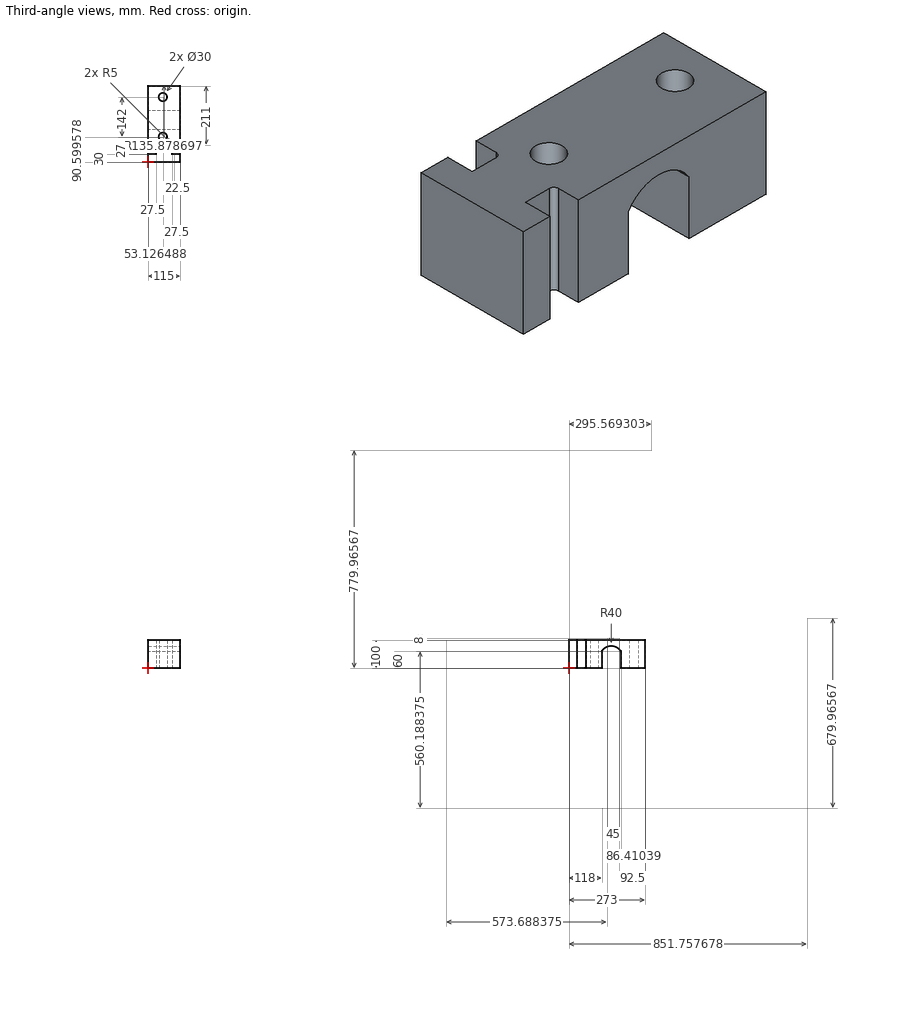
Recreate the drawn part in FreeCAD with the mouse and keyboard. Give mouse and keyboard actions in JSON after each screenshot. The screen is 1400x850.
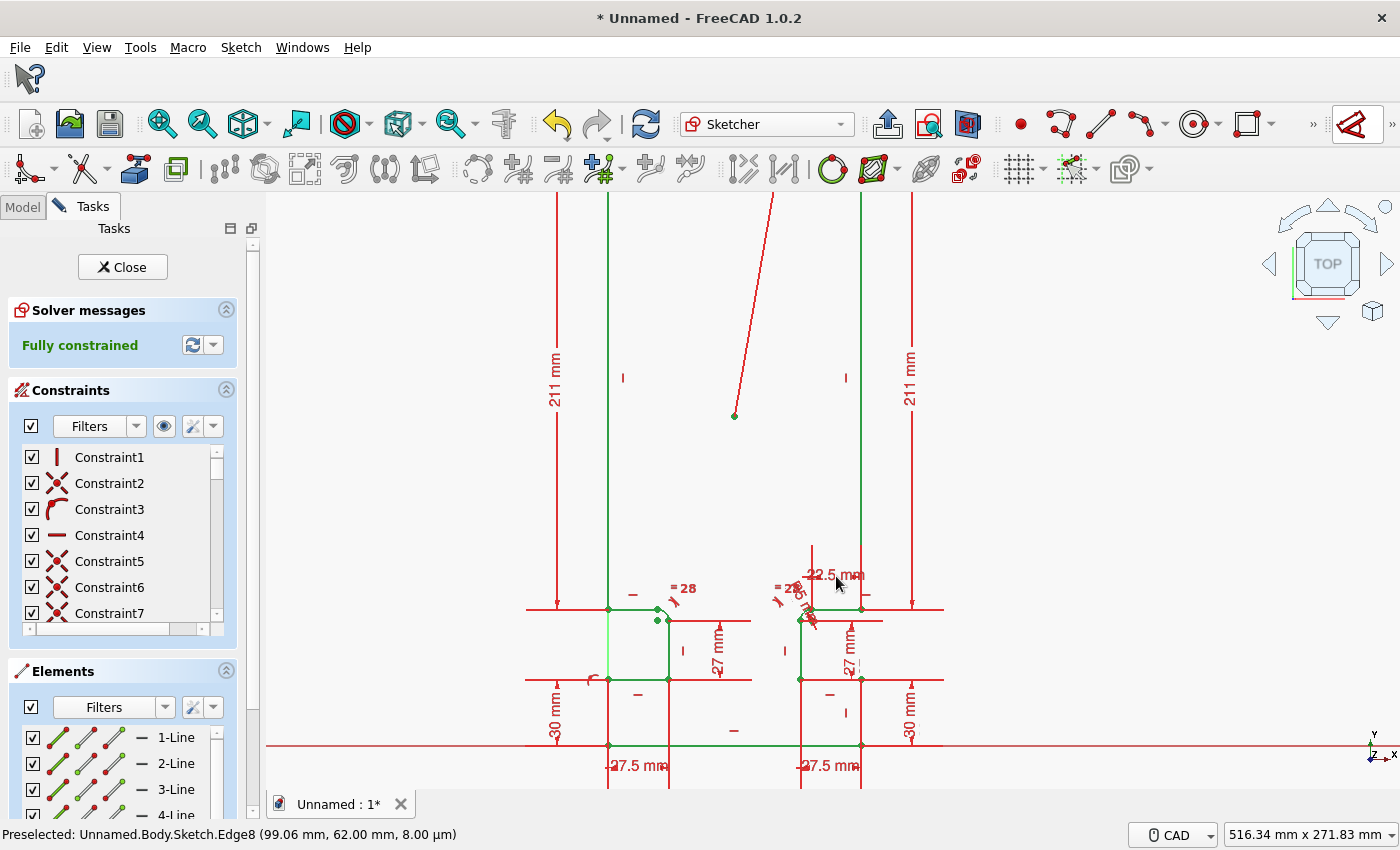
{"action": "left_click", "coordinate": [123, 267]}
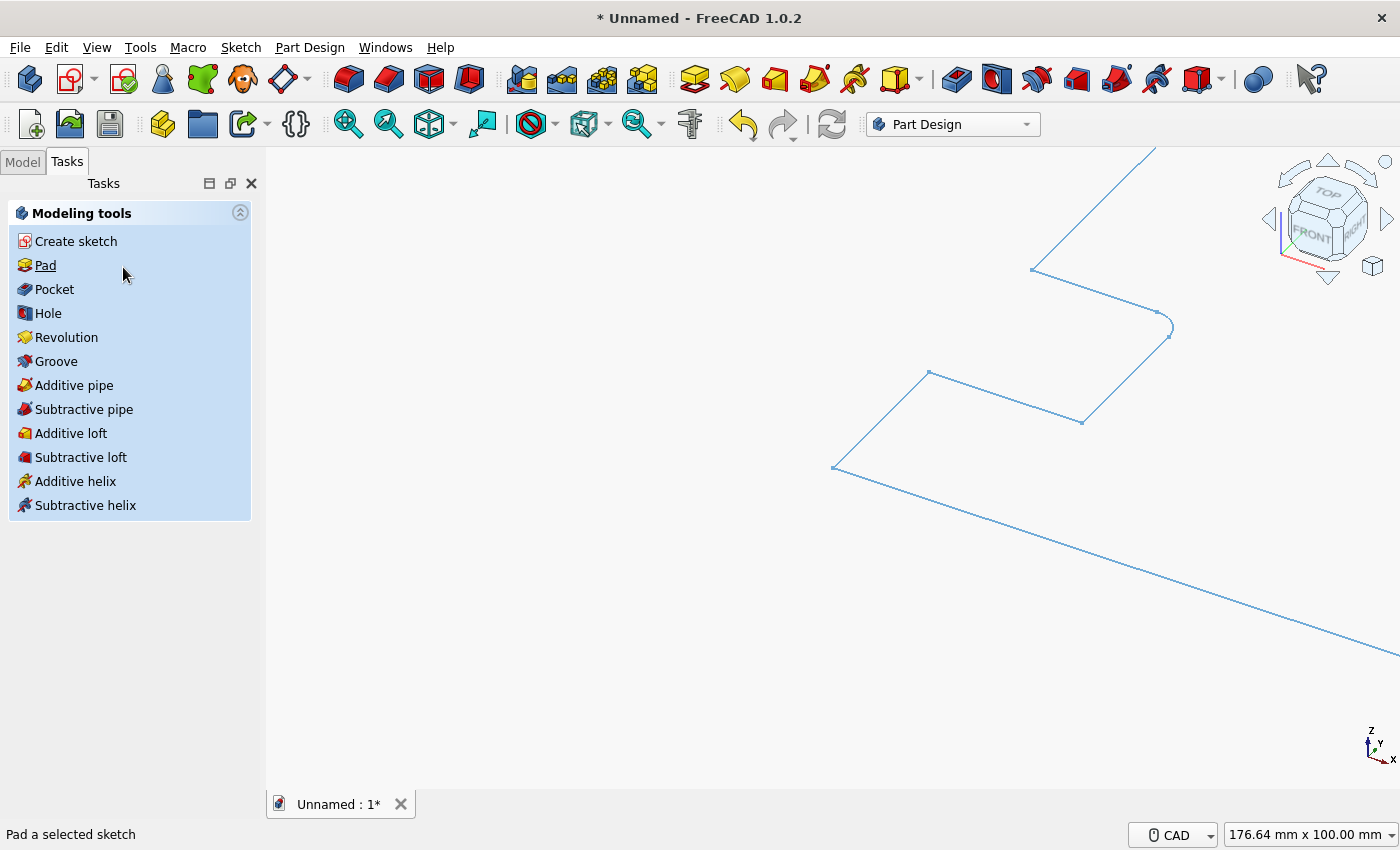
{"action": "left_click", "coordinate": [696, 80]}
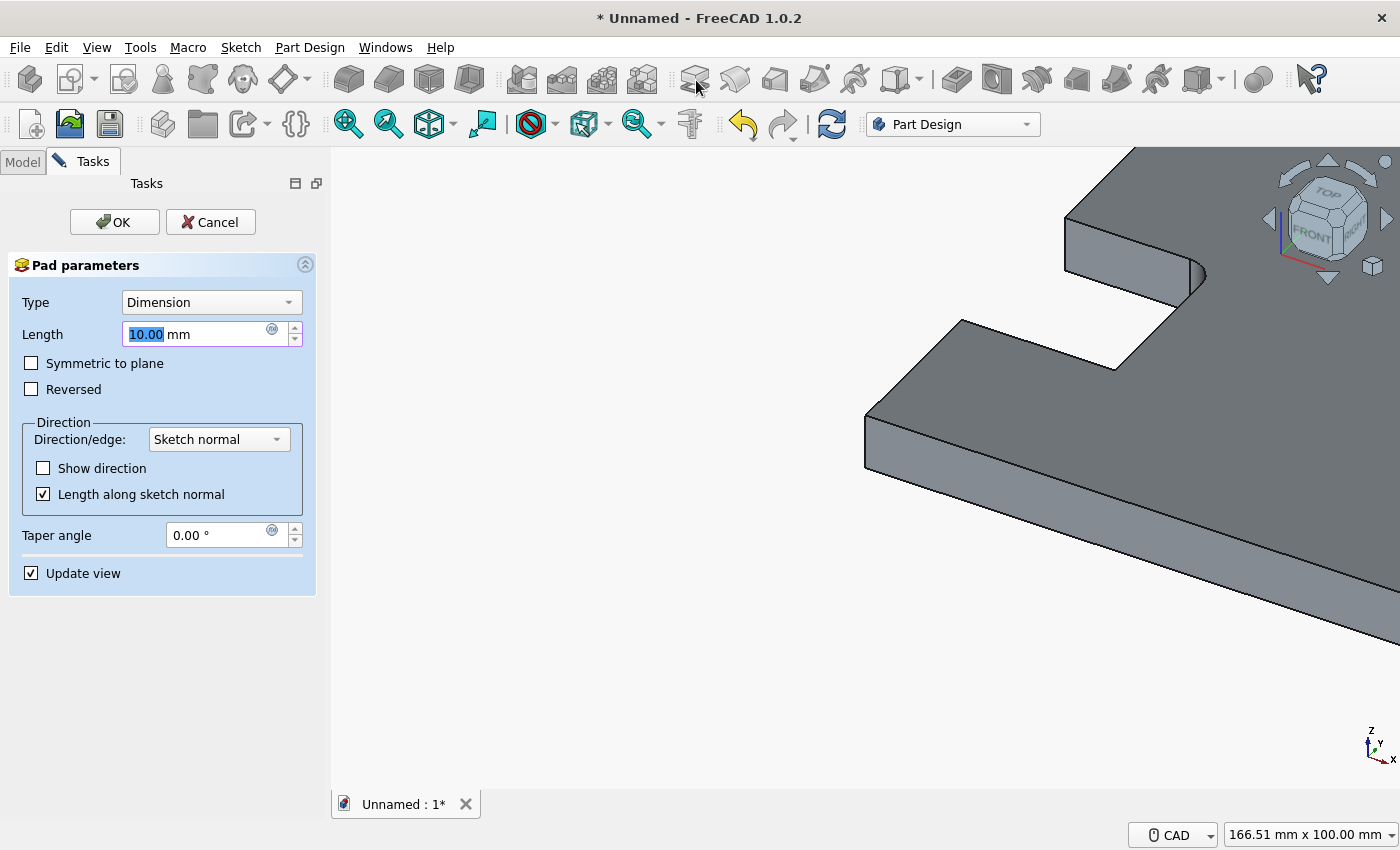
{"action": "type", "text": "100"}
{"action": "key", "text": "Tab"}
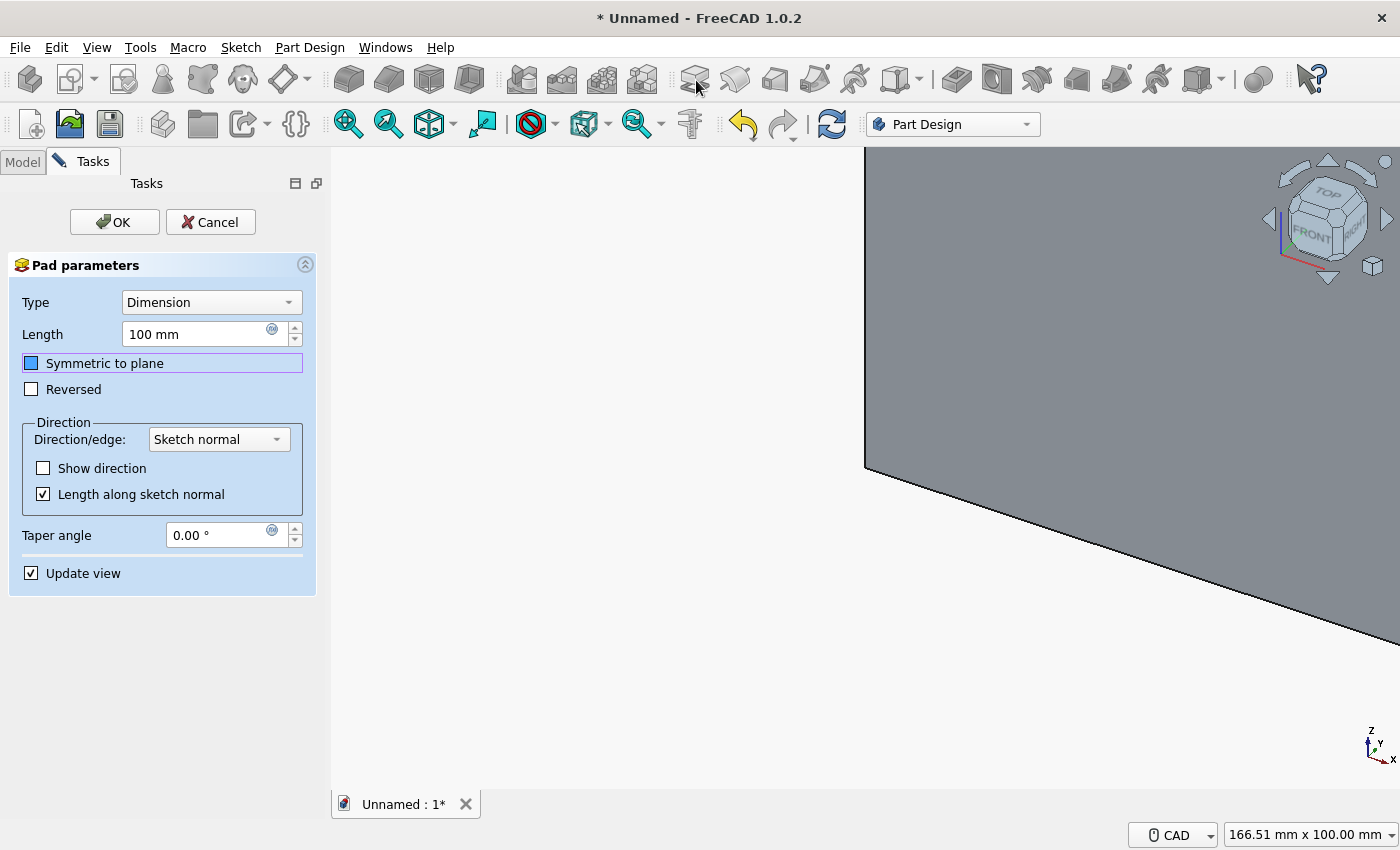
{"action": "left_click", "coordinate": [115, 222]}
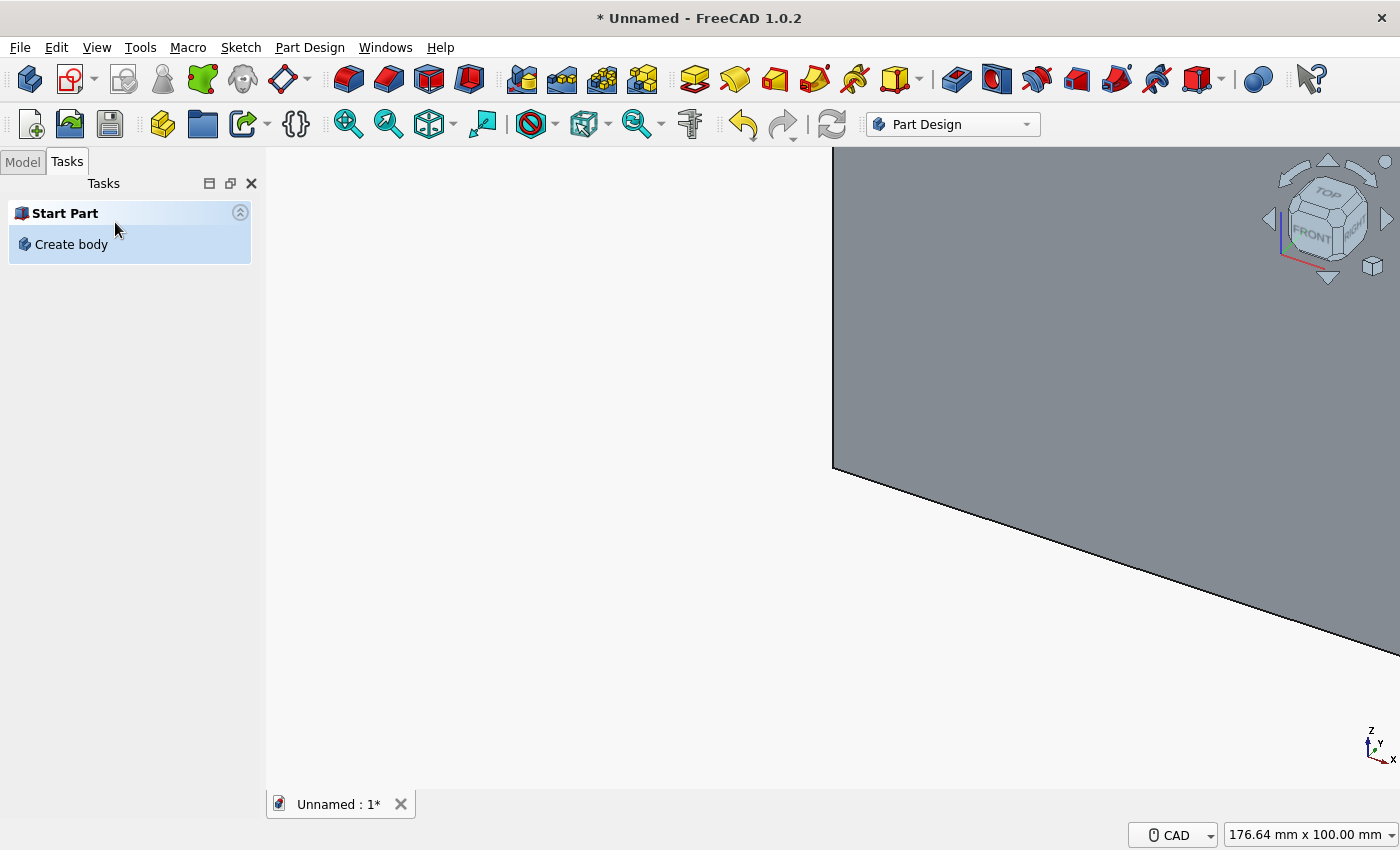
{"action": "key", "text": "v f"}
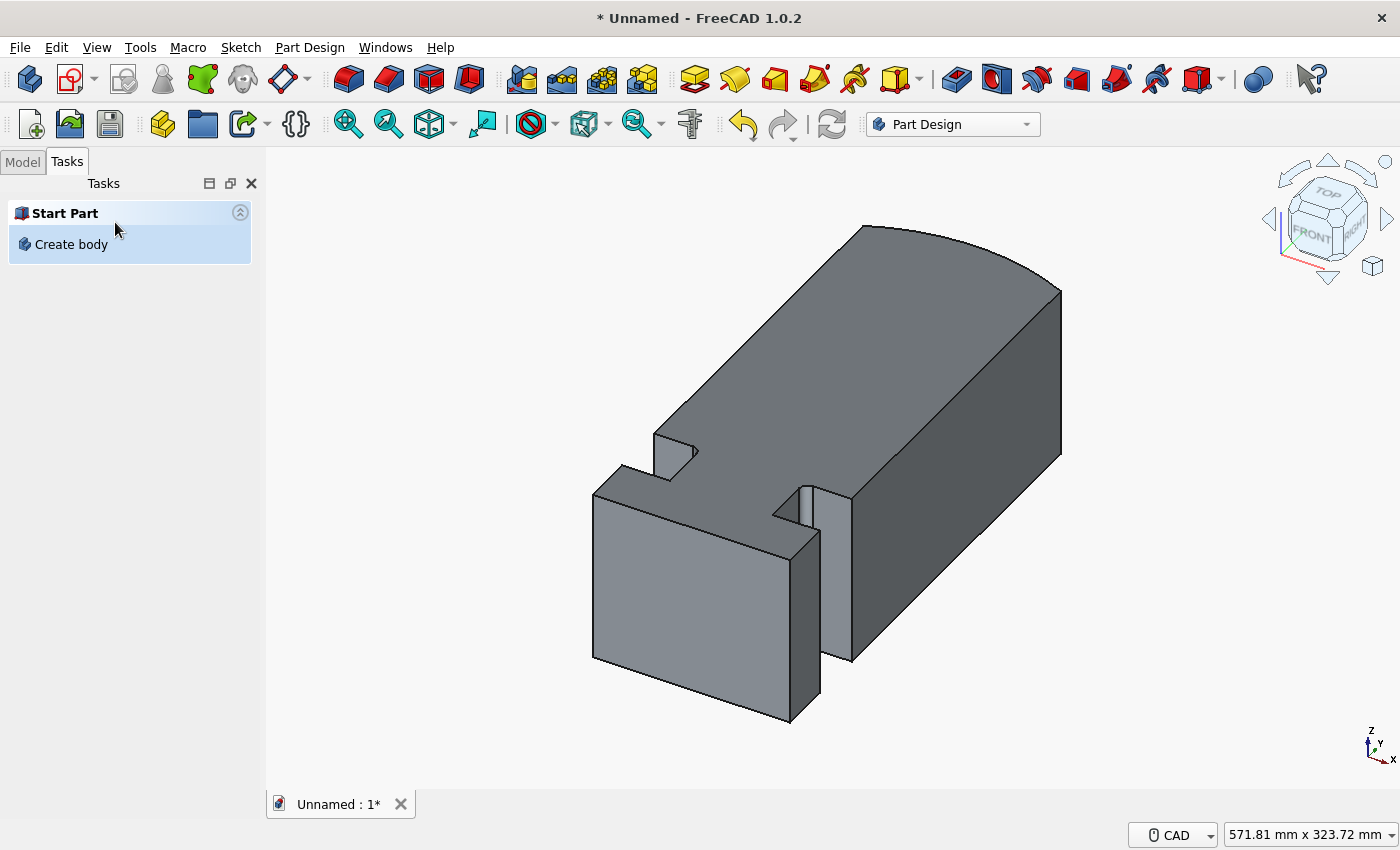
{"action": "left_click", "coordinate": [914, 305]}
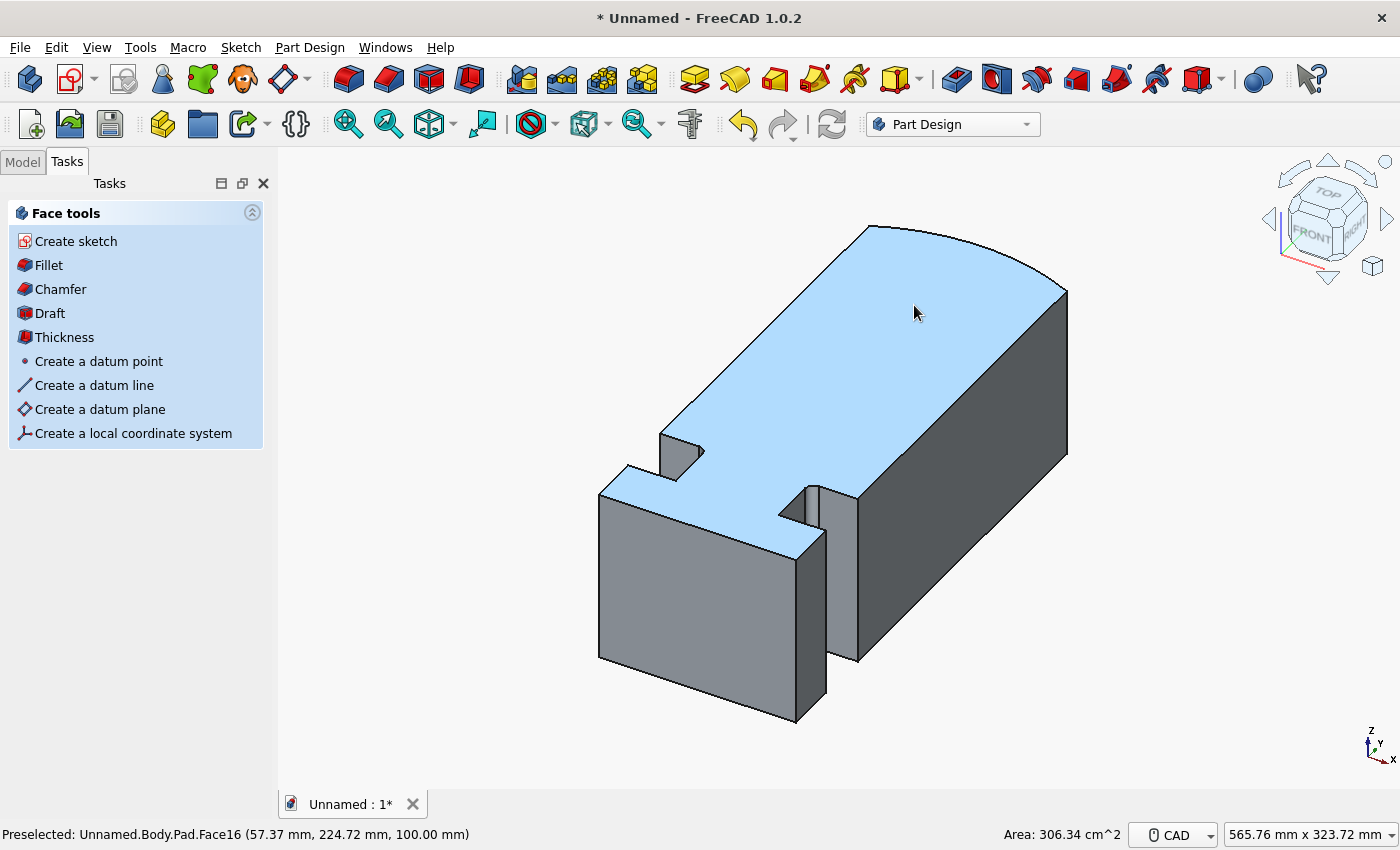
{"action": "left_click", "coordinate": [70, 80]}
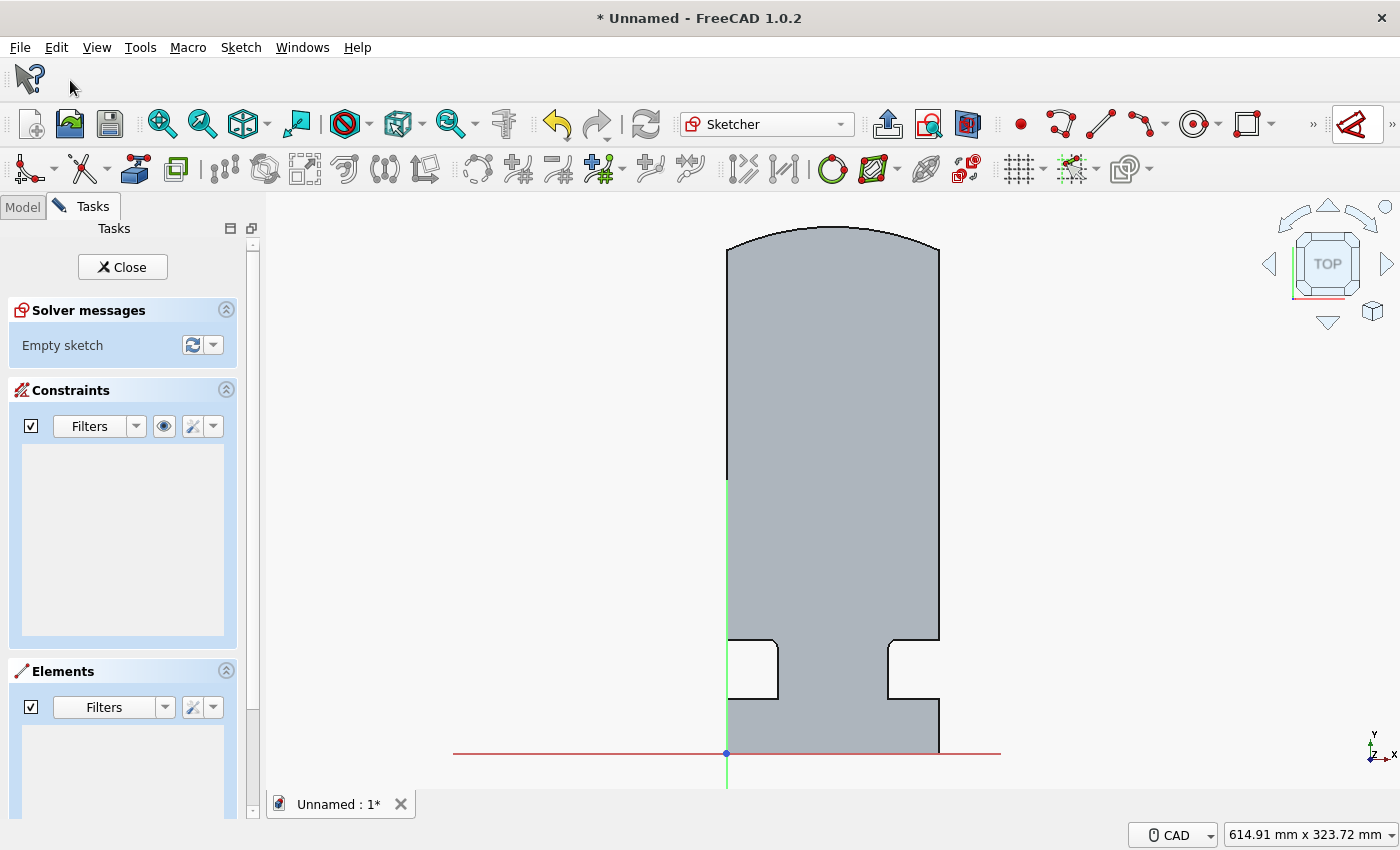
{"action": "scroll", "coordinate": [650, 332], "scroll_direction": "down", "scroll_amount": 1}